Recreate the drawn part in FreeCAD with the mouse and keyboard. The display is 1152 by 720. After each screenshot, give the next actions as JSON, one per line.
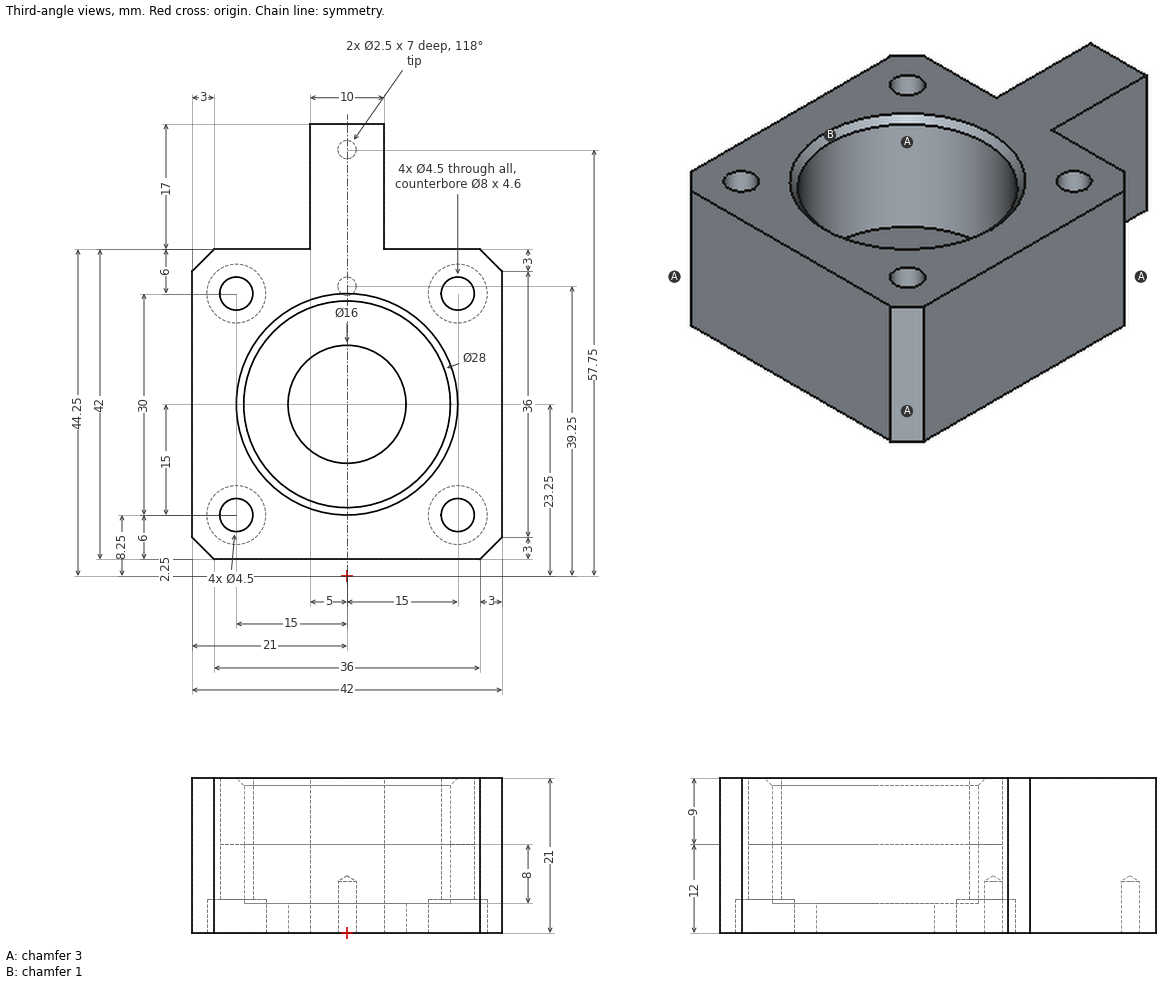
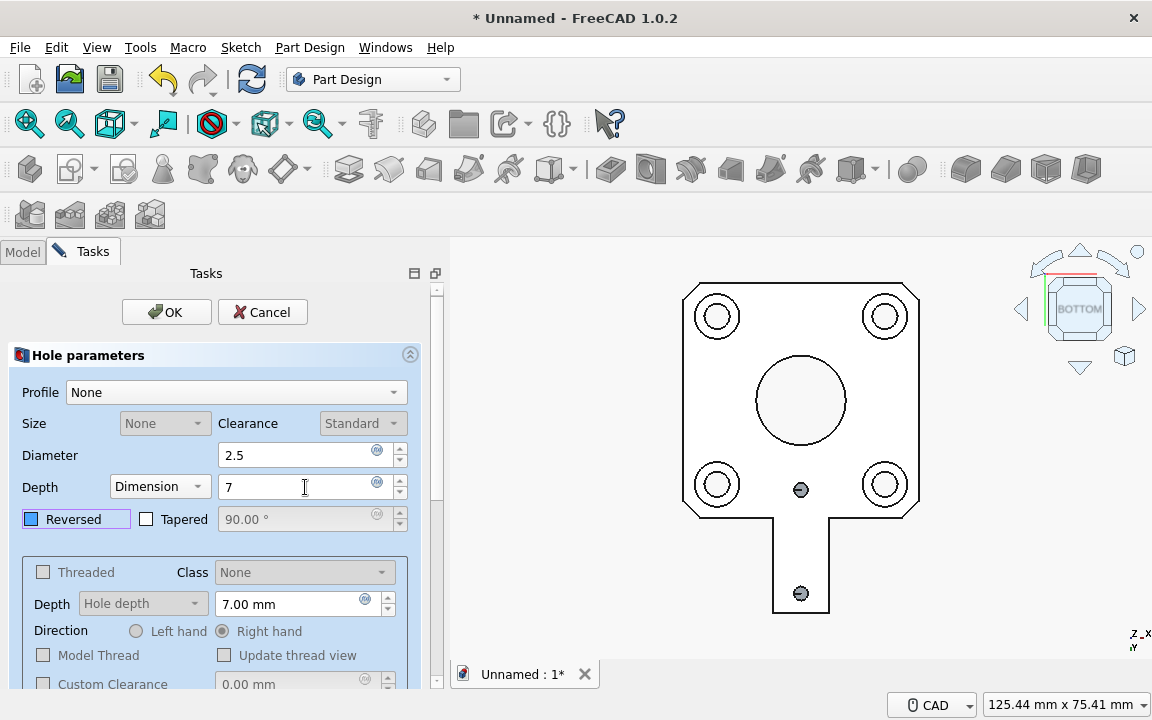
{"action": "left_click", "coordinate": [167, 312]}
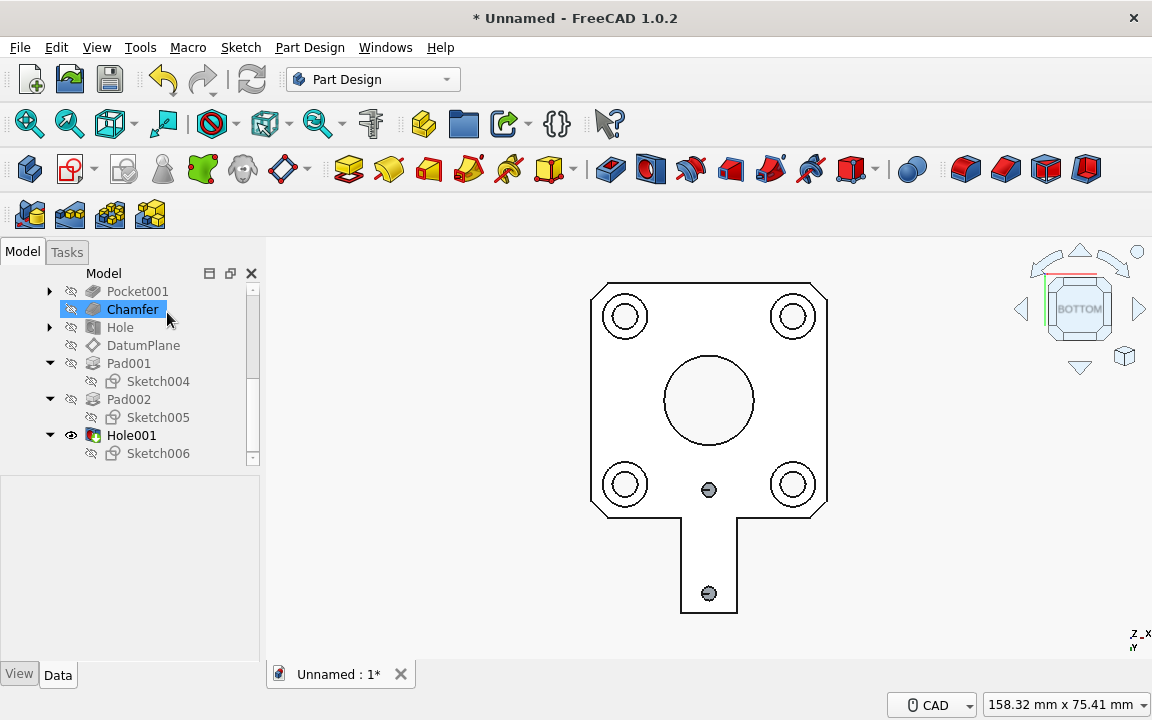
{"action": "key", "text": "0"}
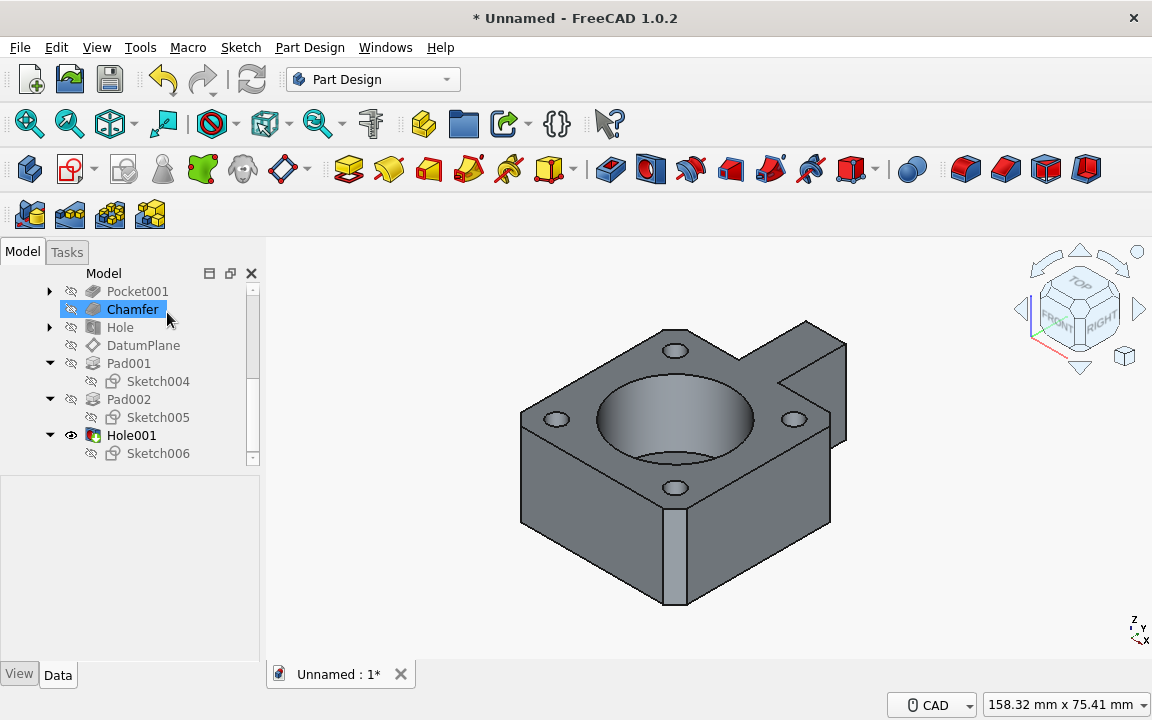
{"action": "left_click", "coordinate": [620, 386]}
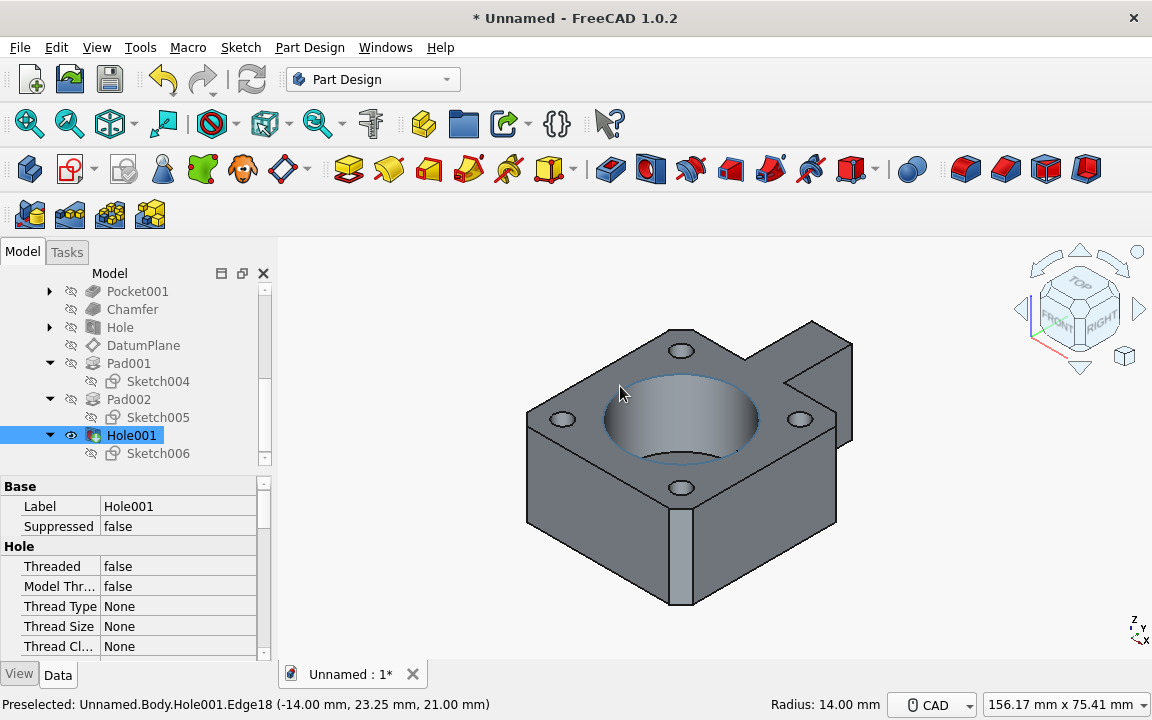
{"action": "left_click", "coordinate": [1006, 170]}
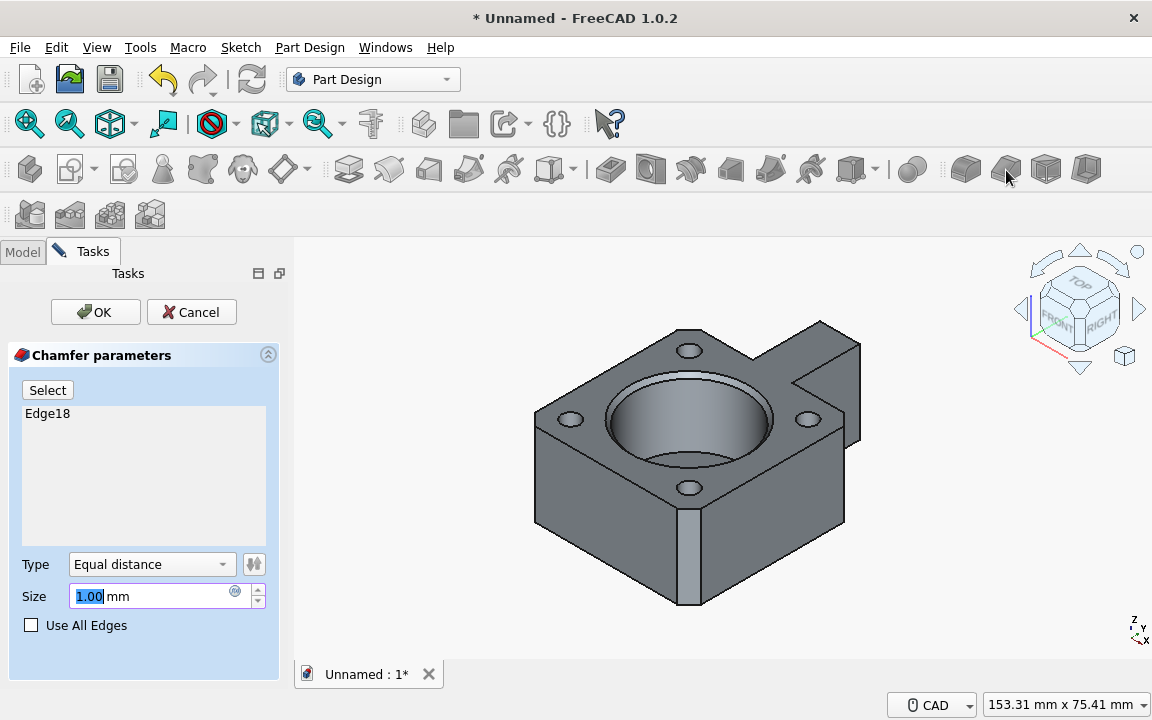
{"action": "type", "text": "1"}
{"action": "key", "text": "Tab"}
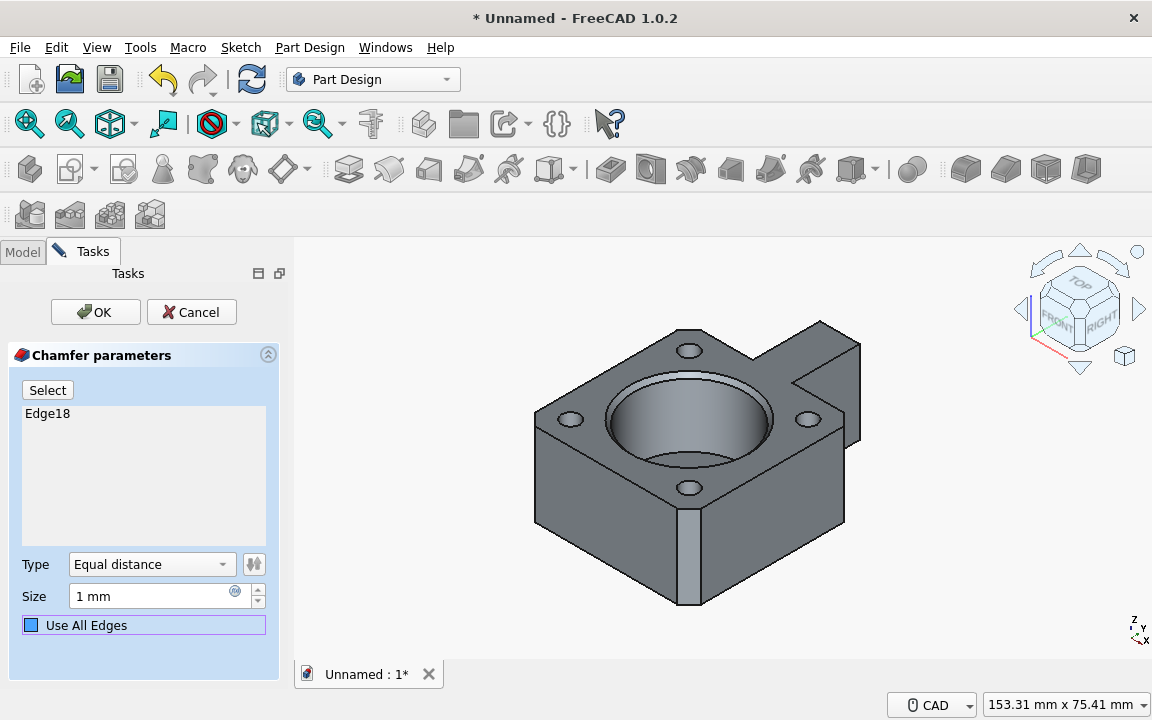
{"action": "left_click", "coordinate": [96, 312]}